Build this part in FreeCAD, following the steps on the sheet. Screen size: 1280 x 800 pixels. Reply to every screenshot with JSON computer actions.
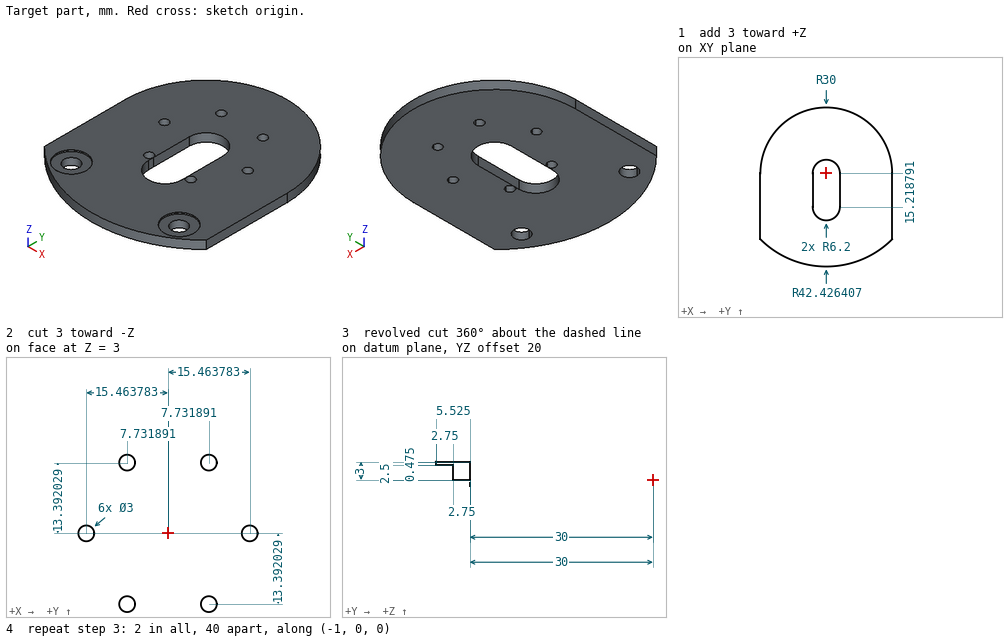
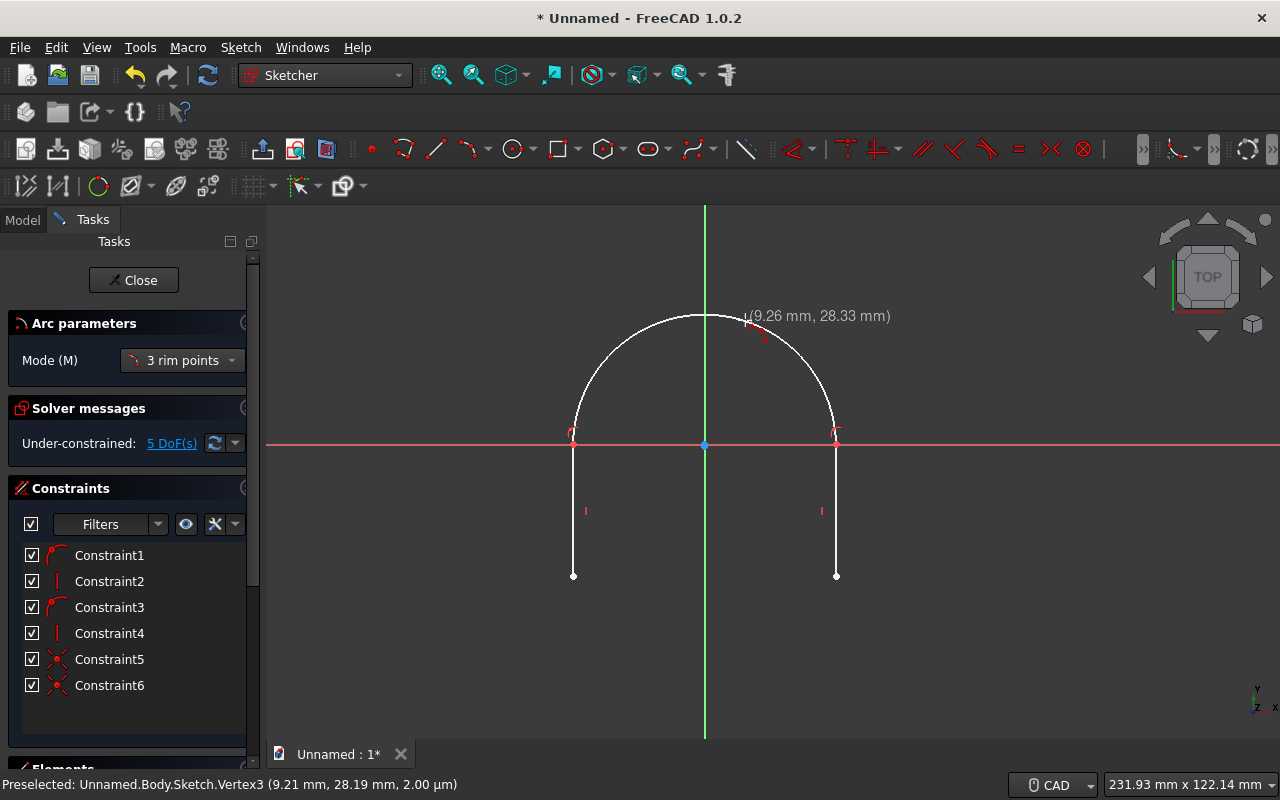
{"action": "left_click", "coordinate": [573, 577]}
{"action": "left_click", "coordinate": [836, 577]}
{"action": "left_click", "coordinate": [675, 628]}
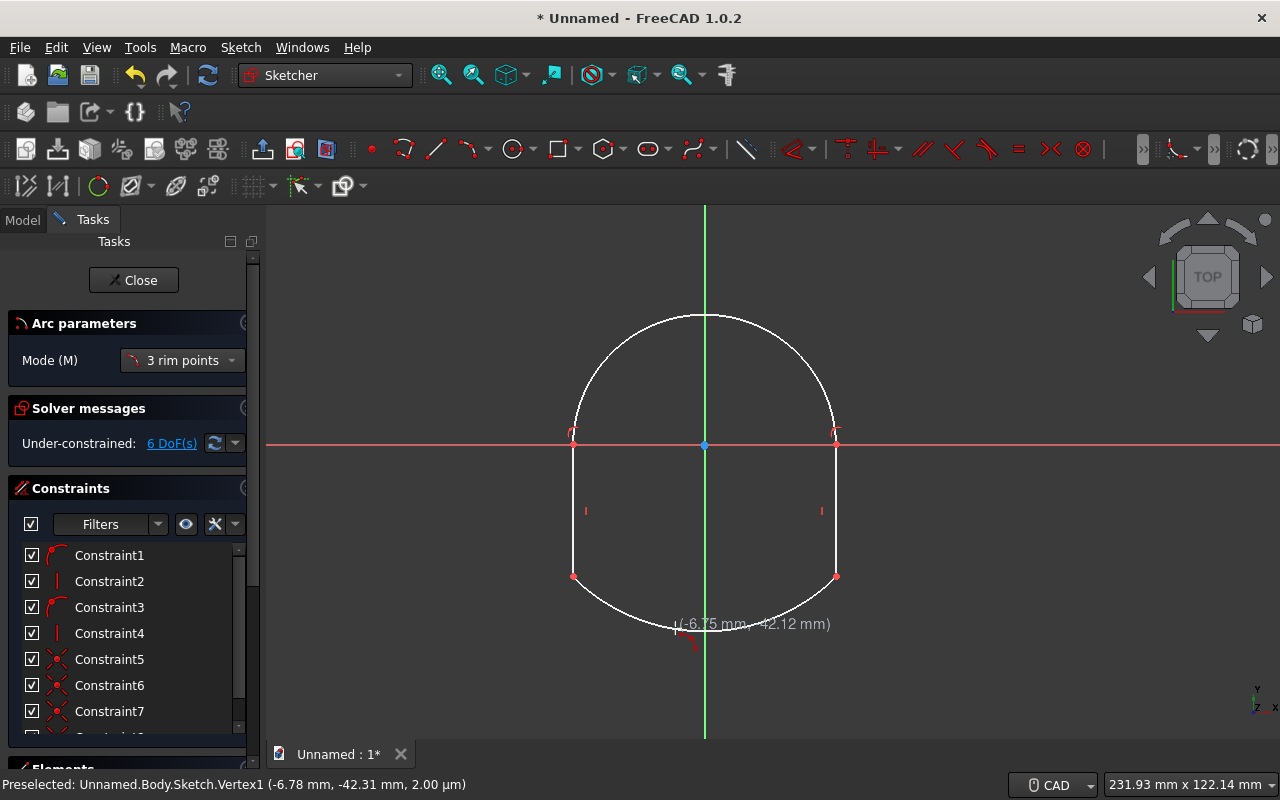
{"action": "key", "text": "g s"}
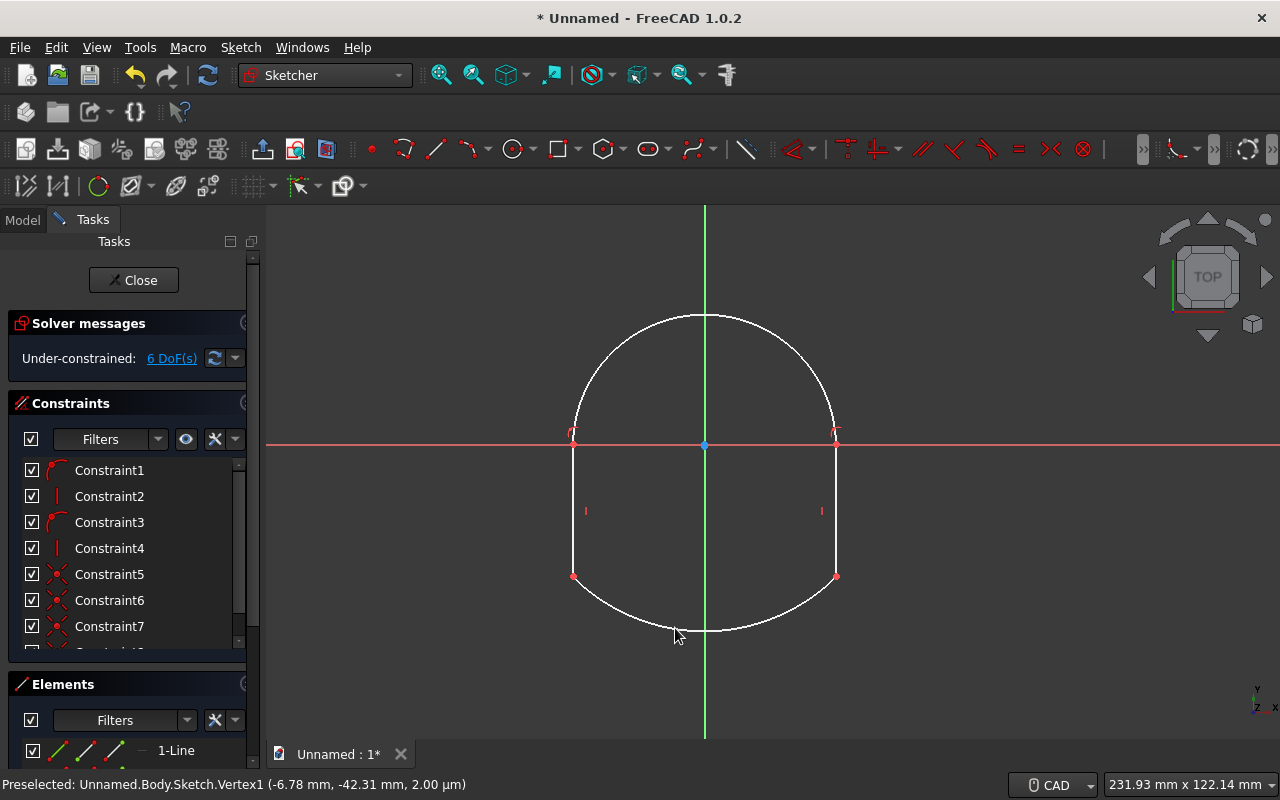
{"action": "left_click", "coordinate": [705, 445]}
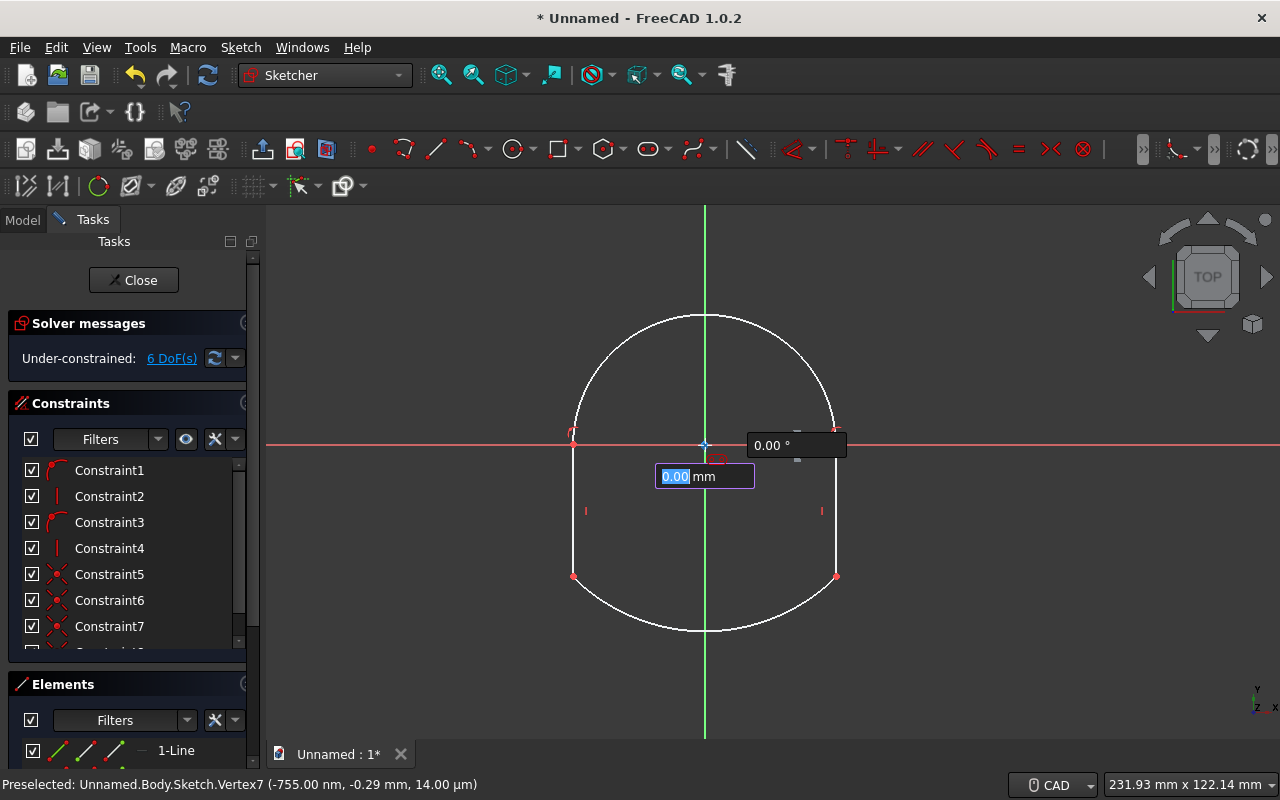
{"action": "left_click", "coordinate": [714, 511]}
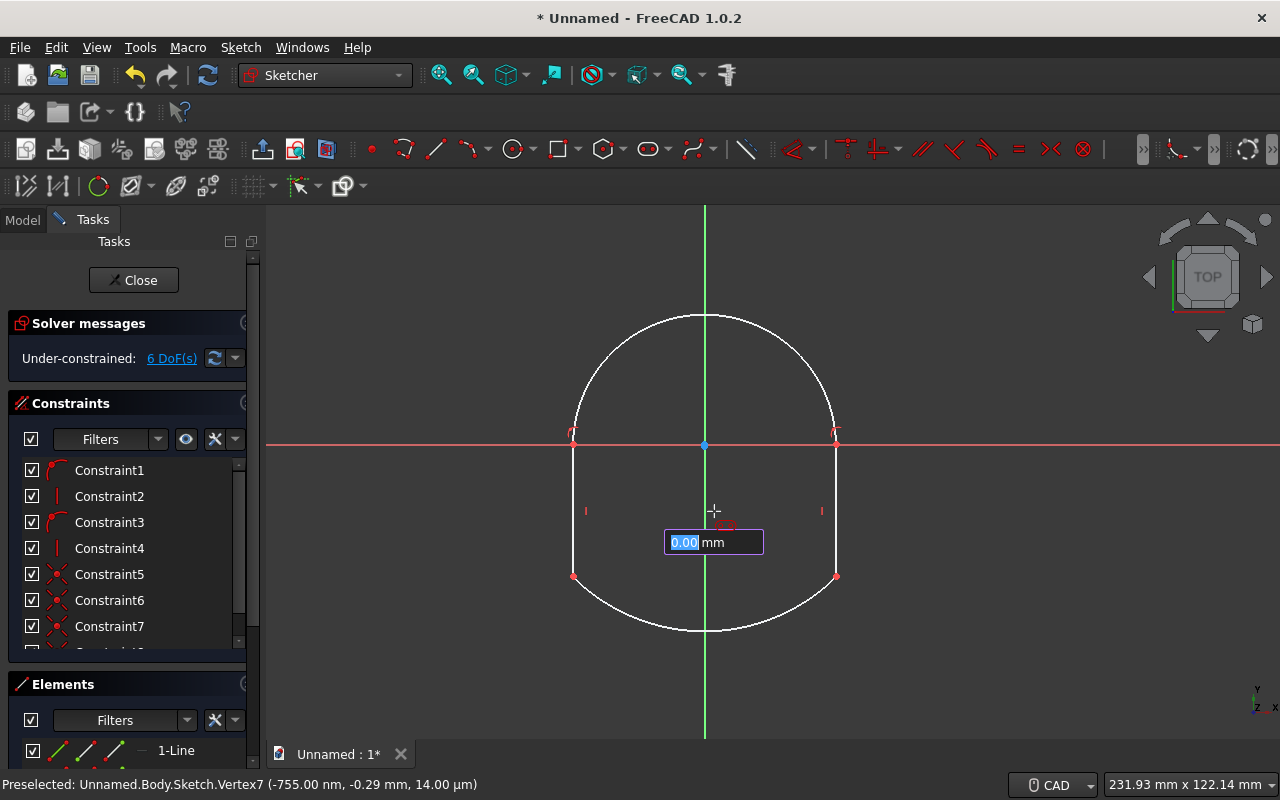
{"action": "left_click", "coordinate": [732, 478]}
{"action": "key", "text": "Escape"}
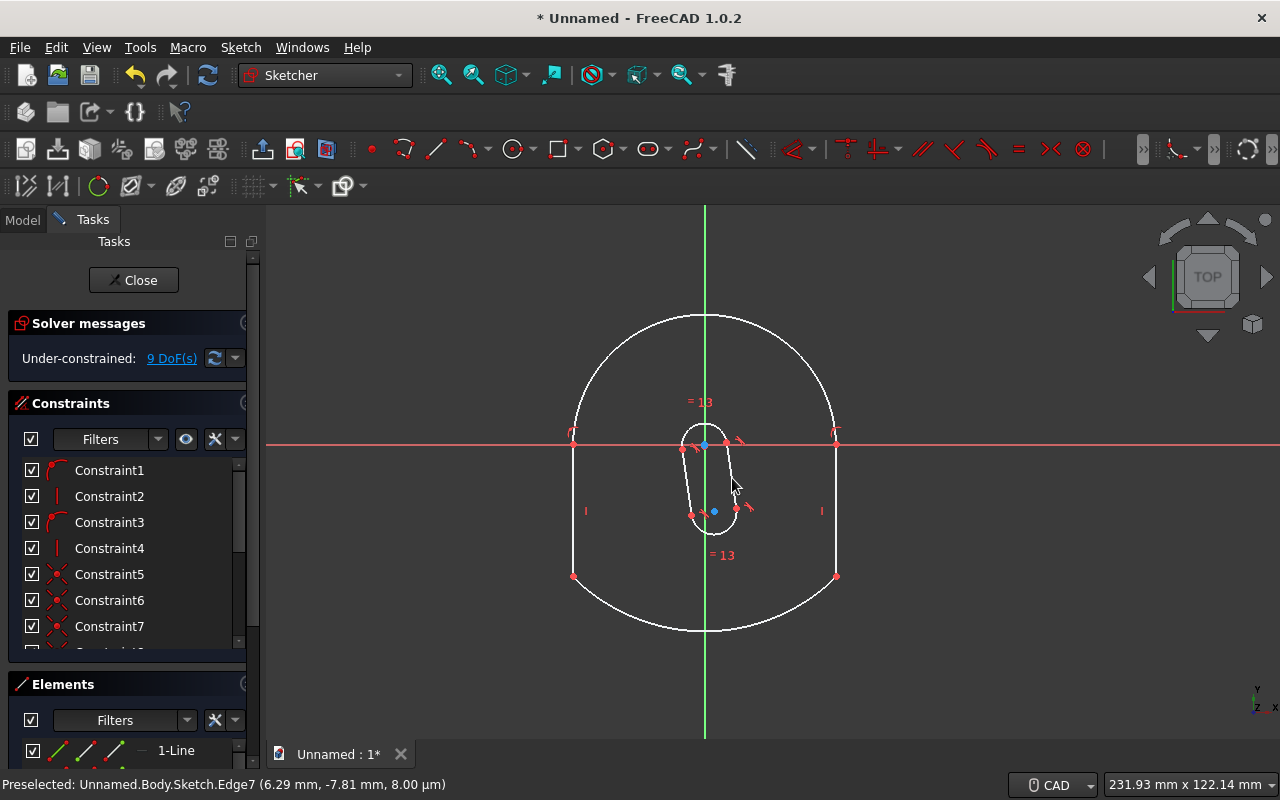
{"action": "left_click", "coordinate": [730, 463]}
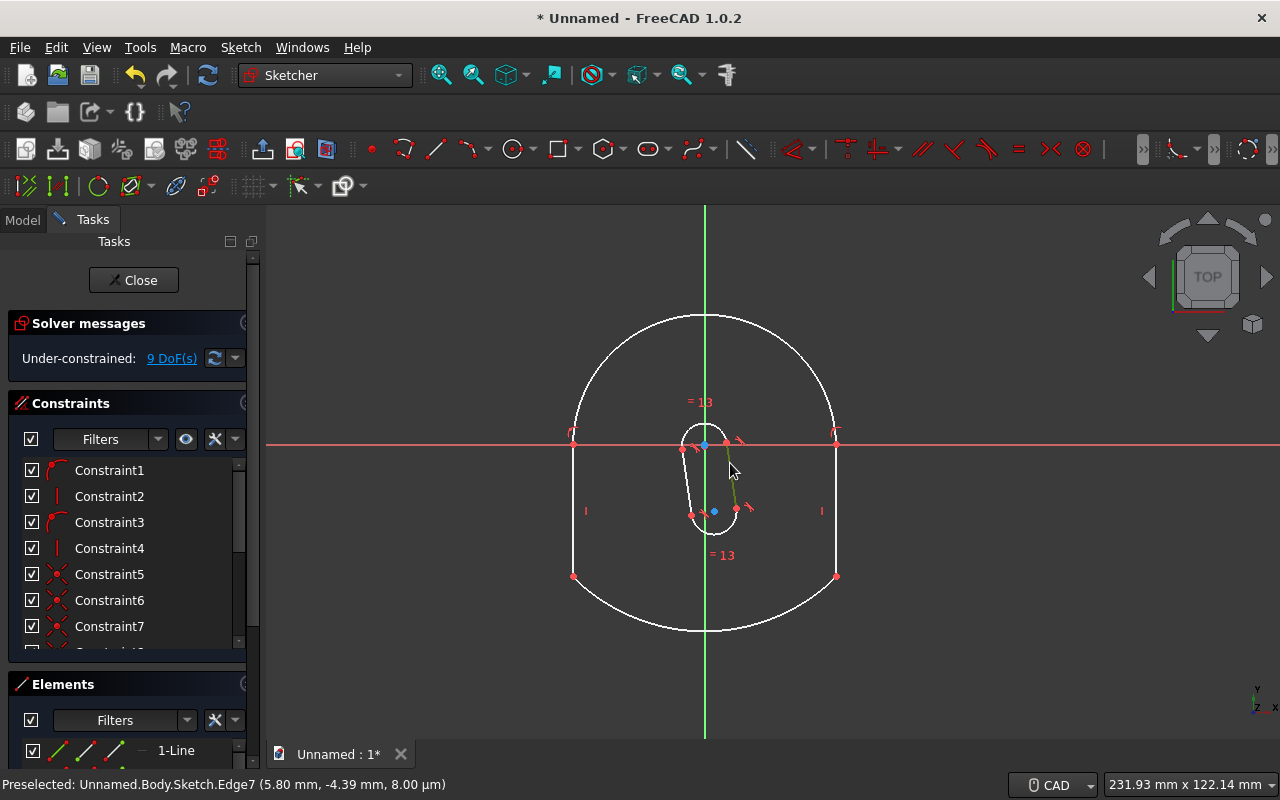
{"action": "key", "text": "v"}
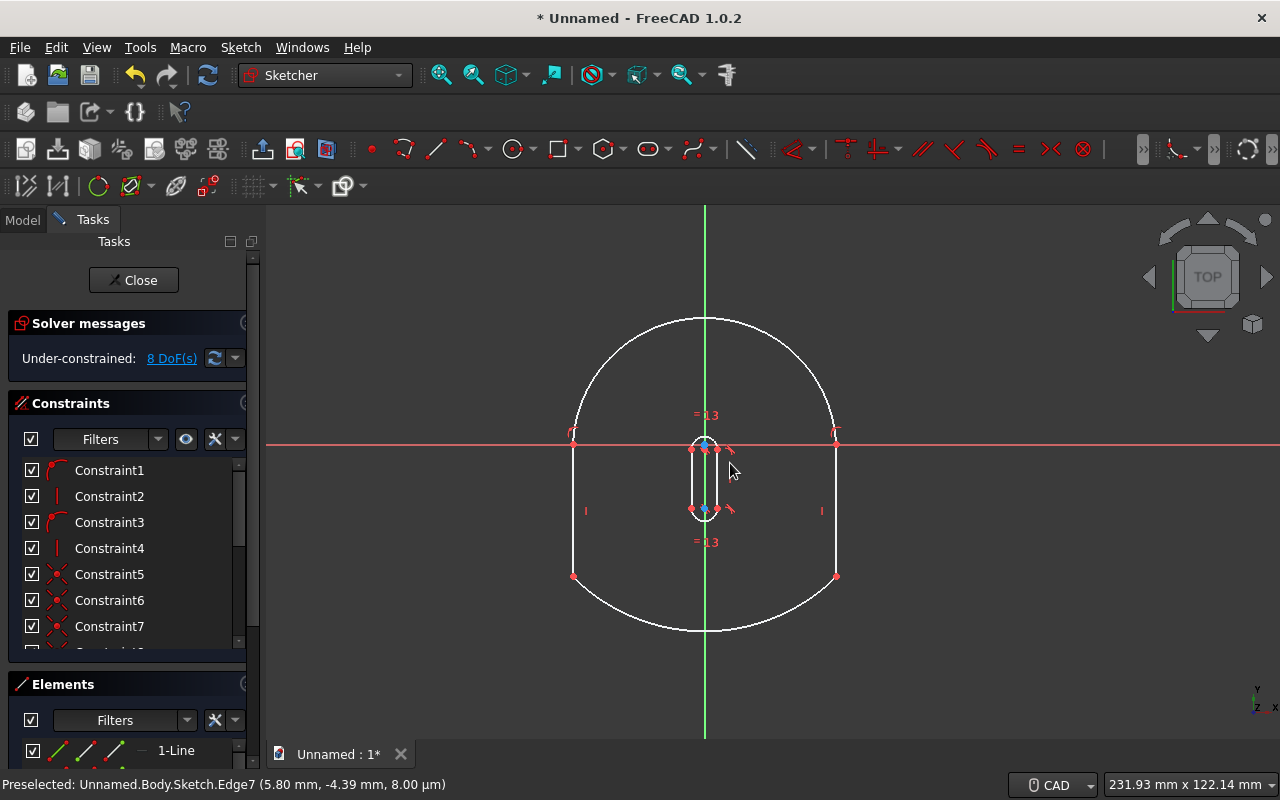
{"action": "left_click", "coordinate": [780, 342]}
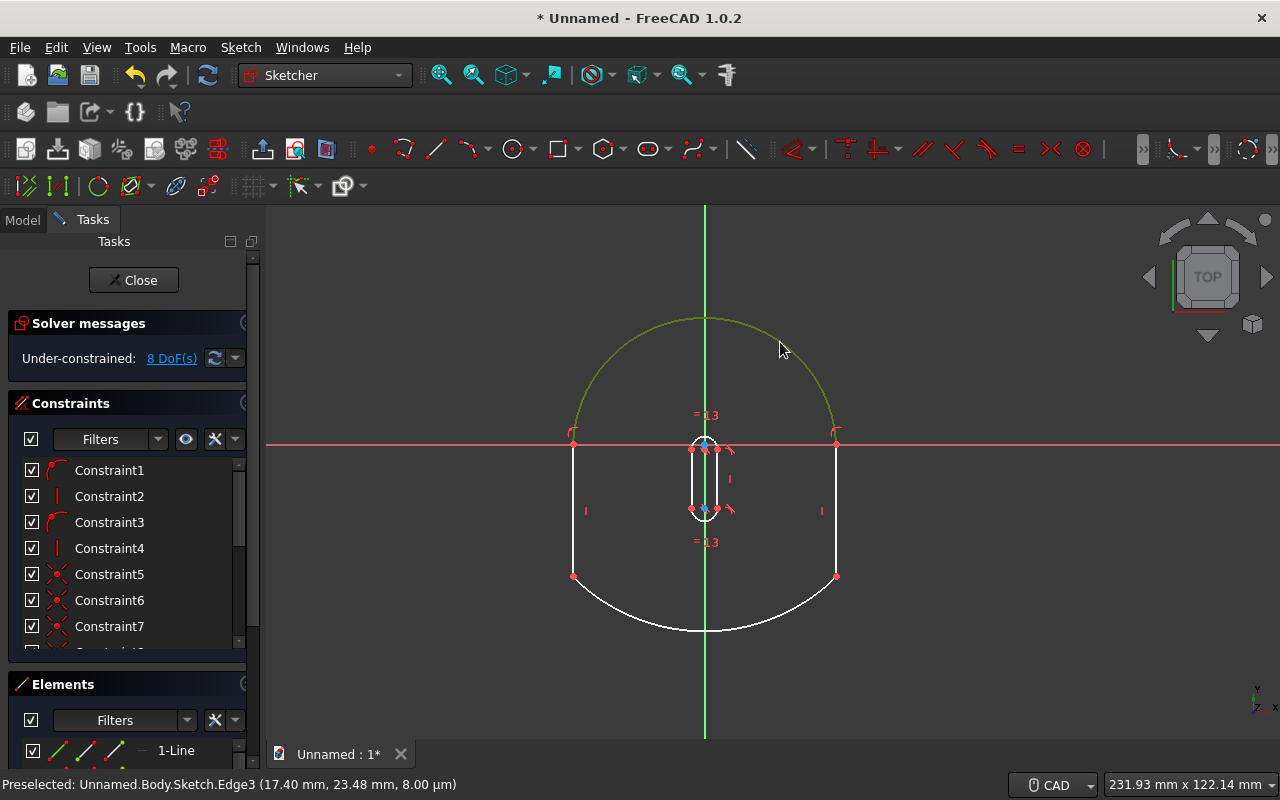
{"action": "left_click", "coordinate": [647, 622]}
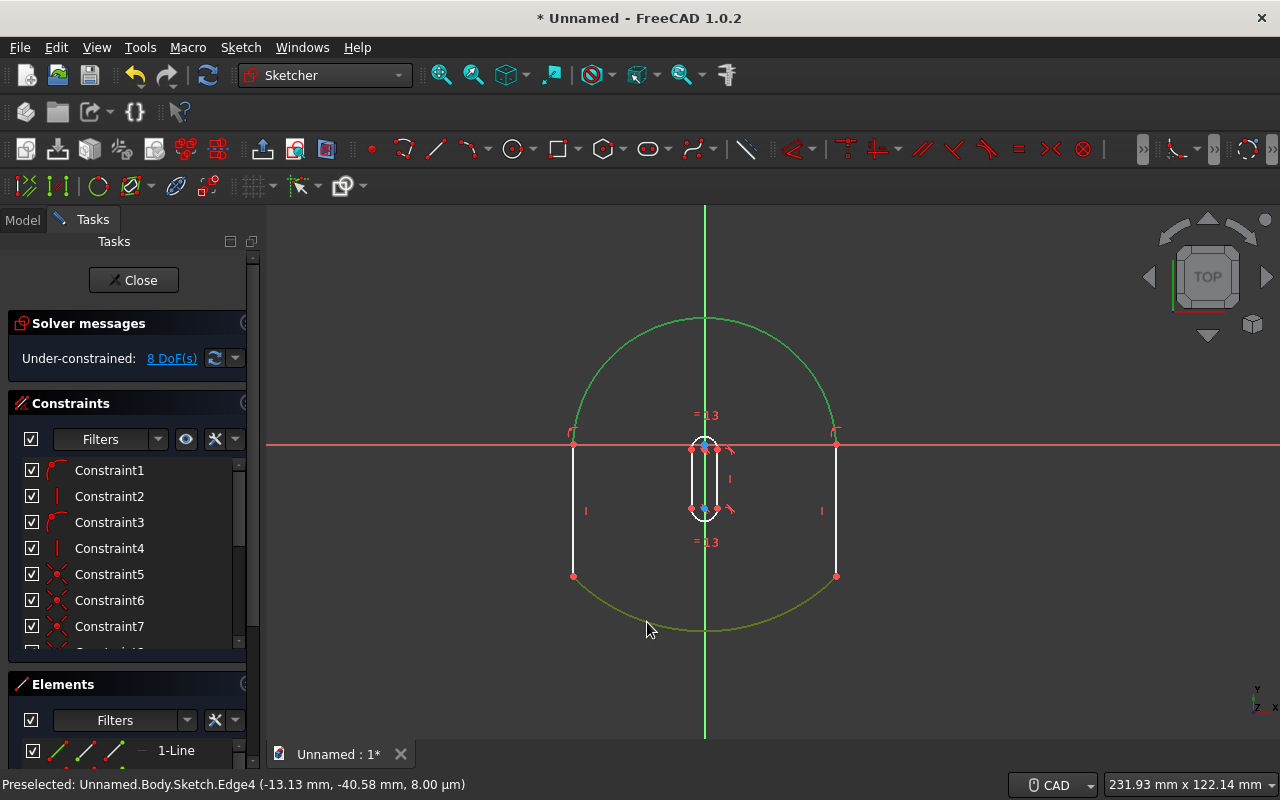
{"action": "key", "text": "c"}